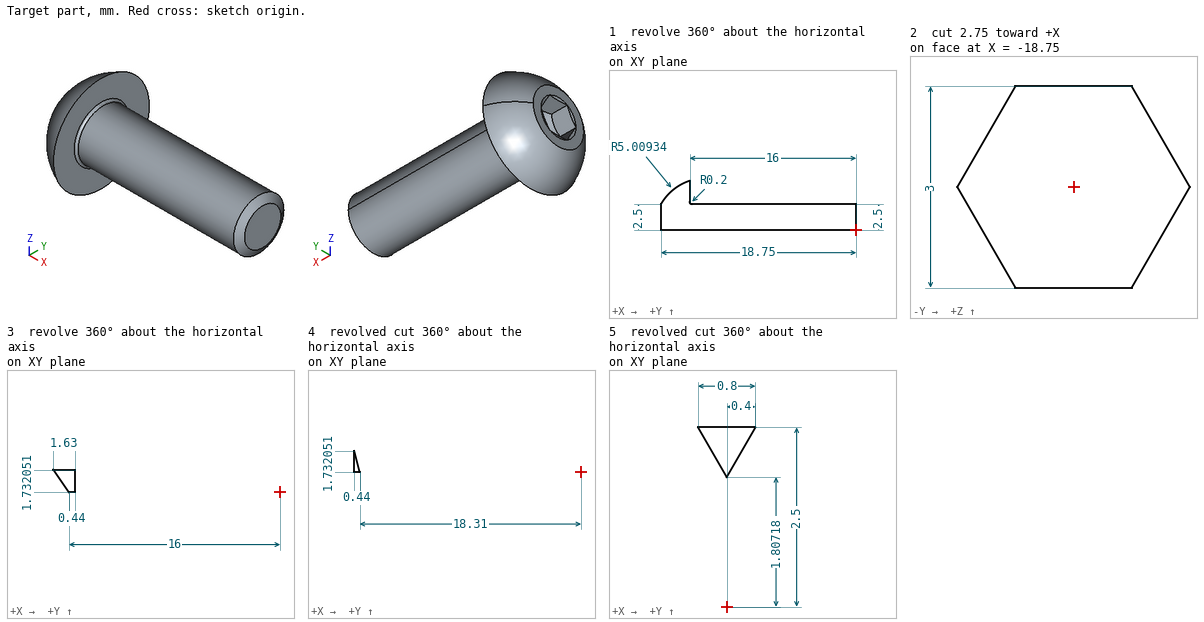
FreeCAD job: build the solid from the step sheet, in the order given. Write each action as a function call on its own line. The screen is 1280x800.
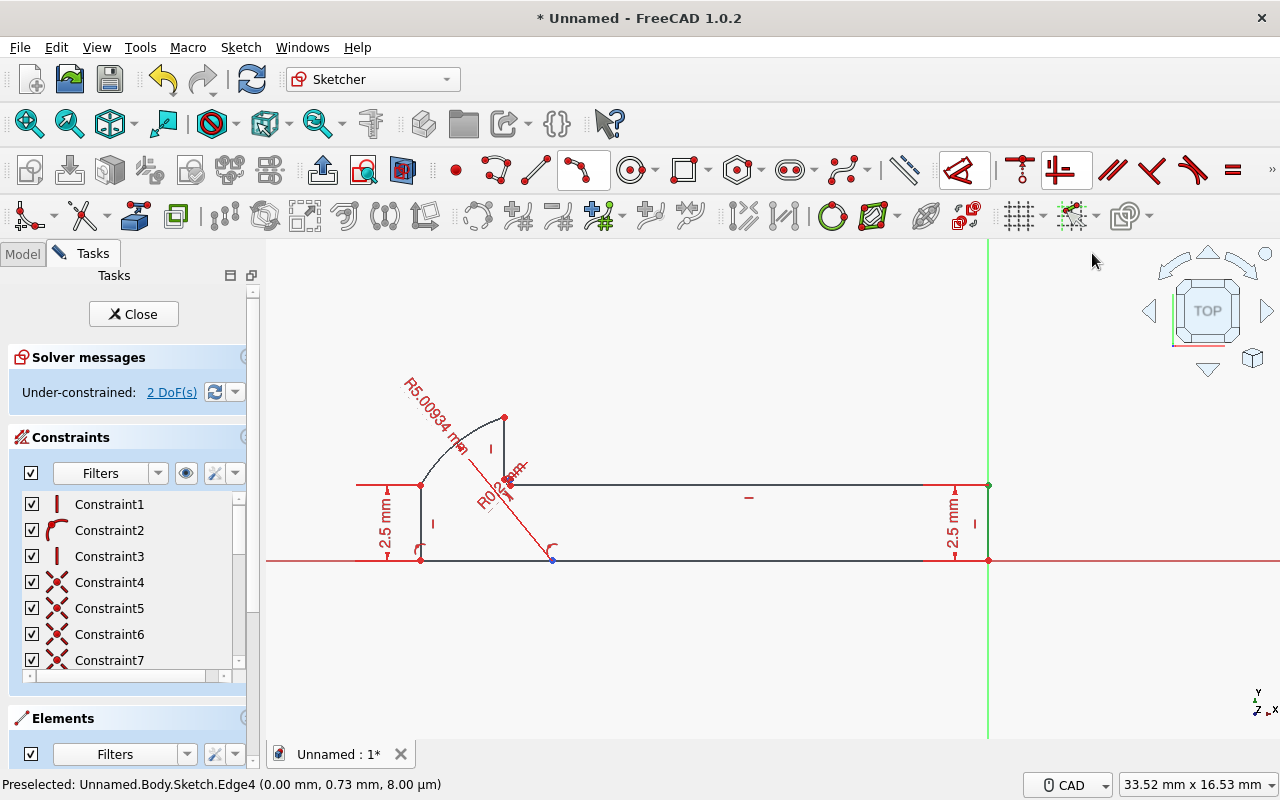
scroll(504, 479, up, 4)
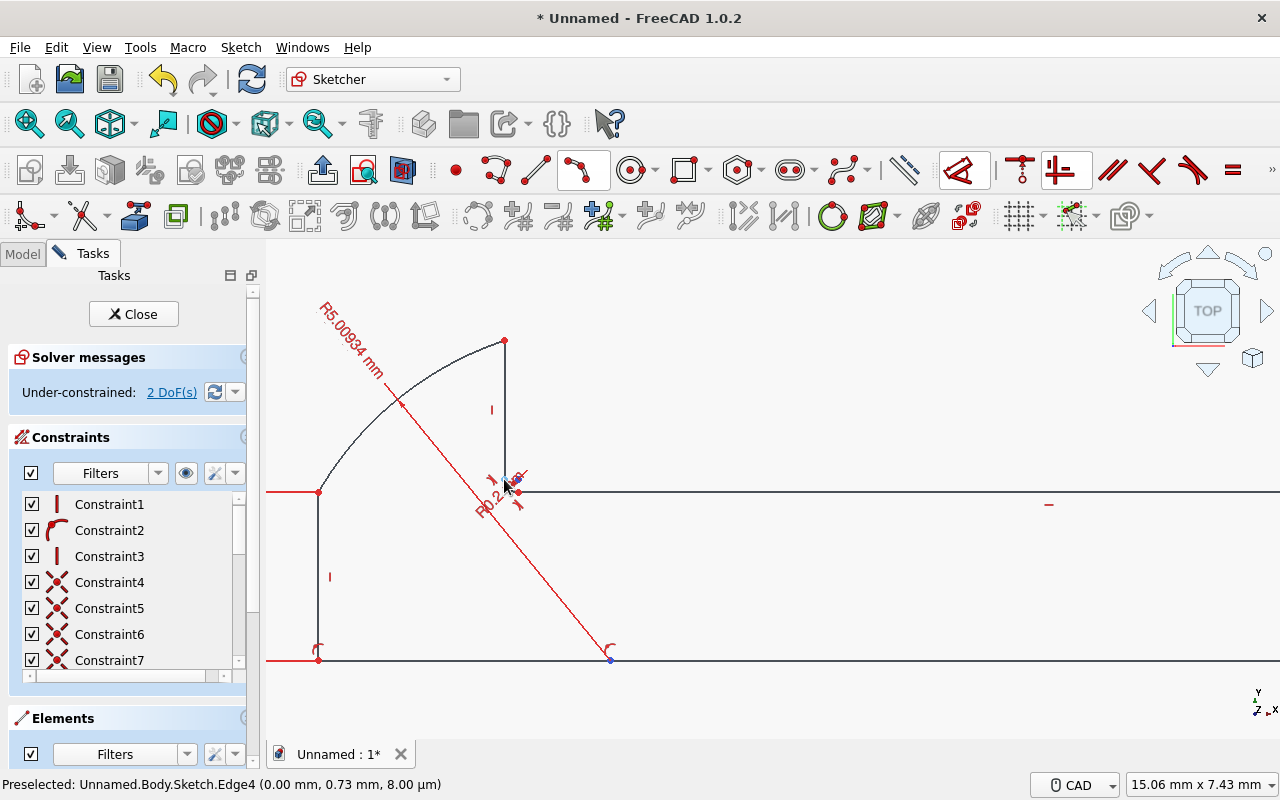
click(505, 479)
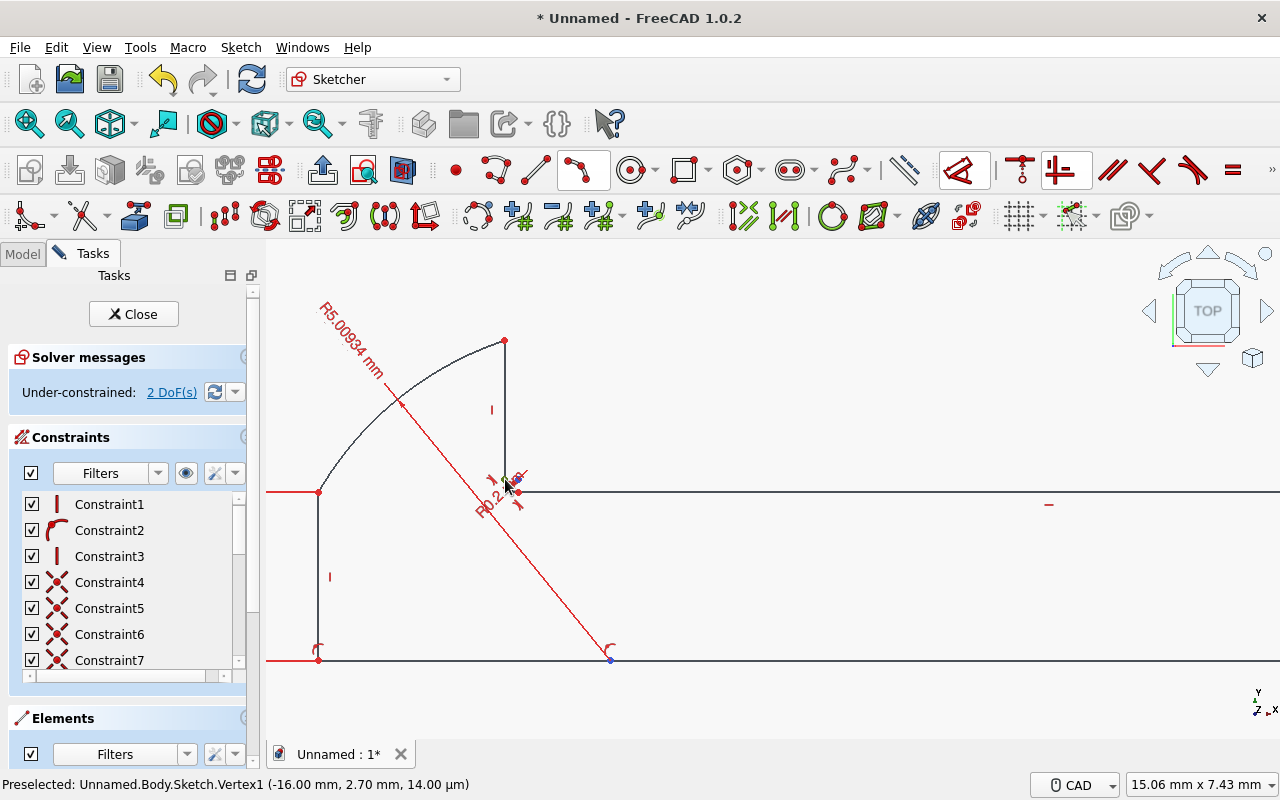
key(l)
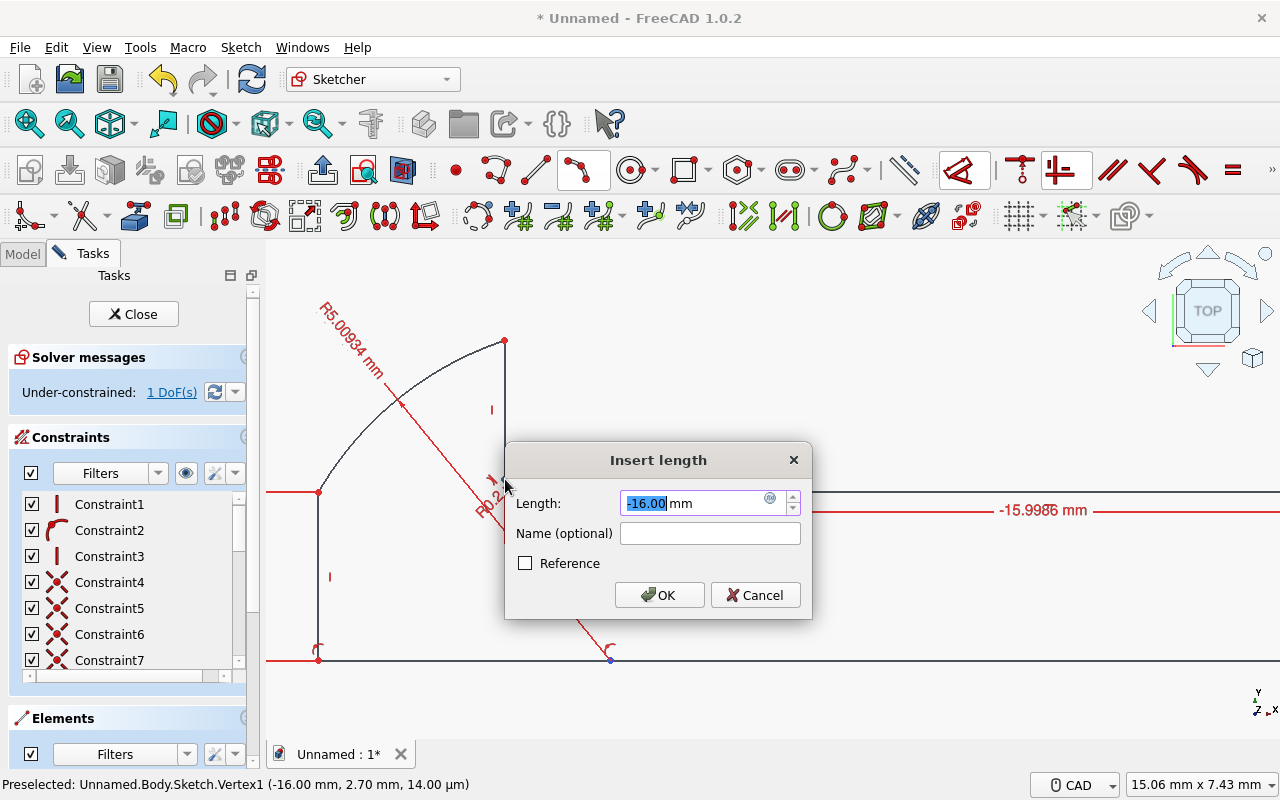
text(-16)
key(Return)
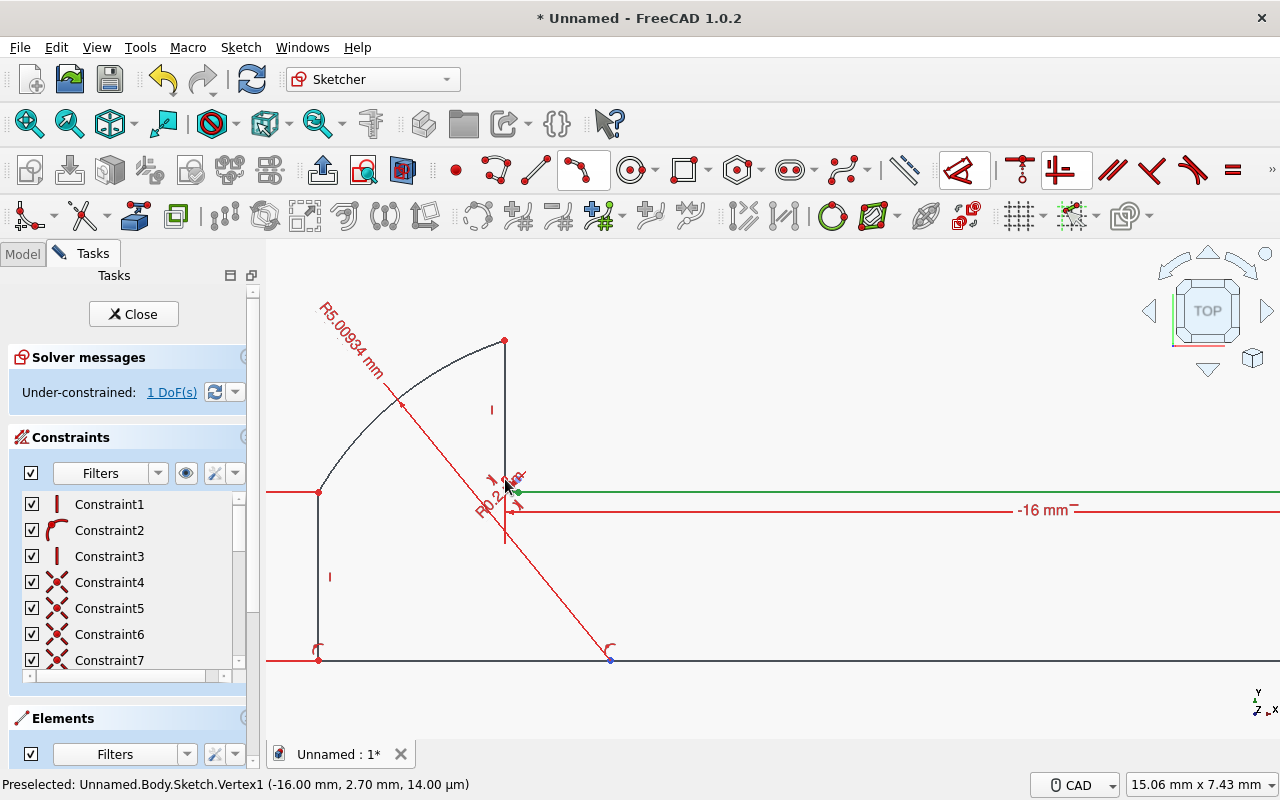
click(697, 661)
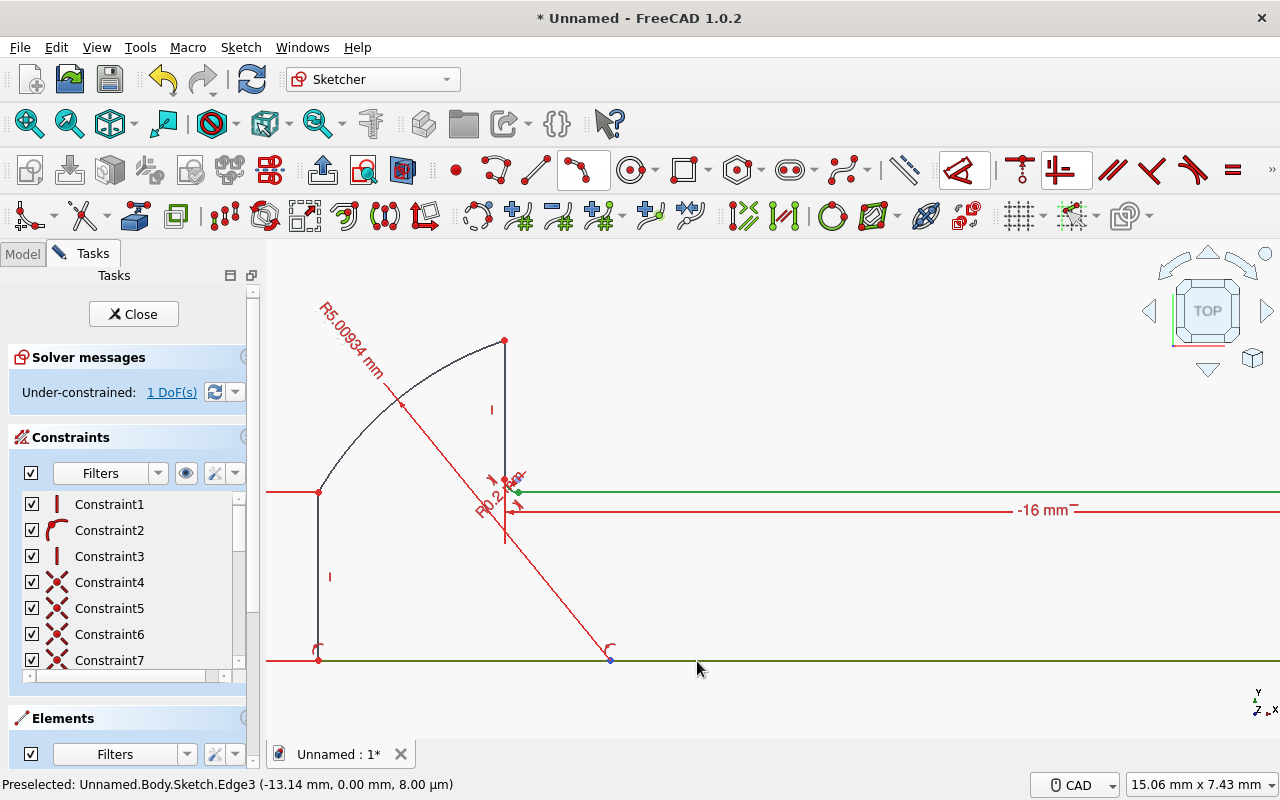
key(l)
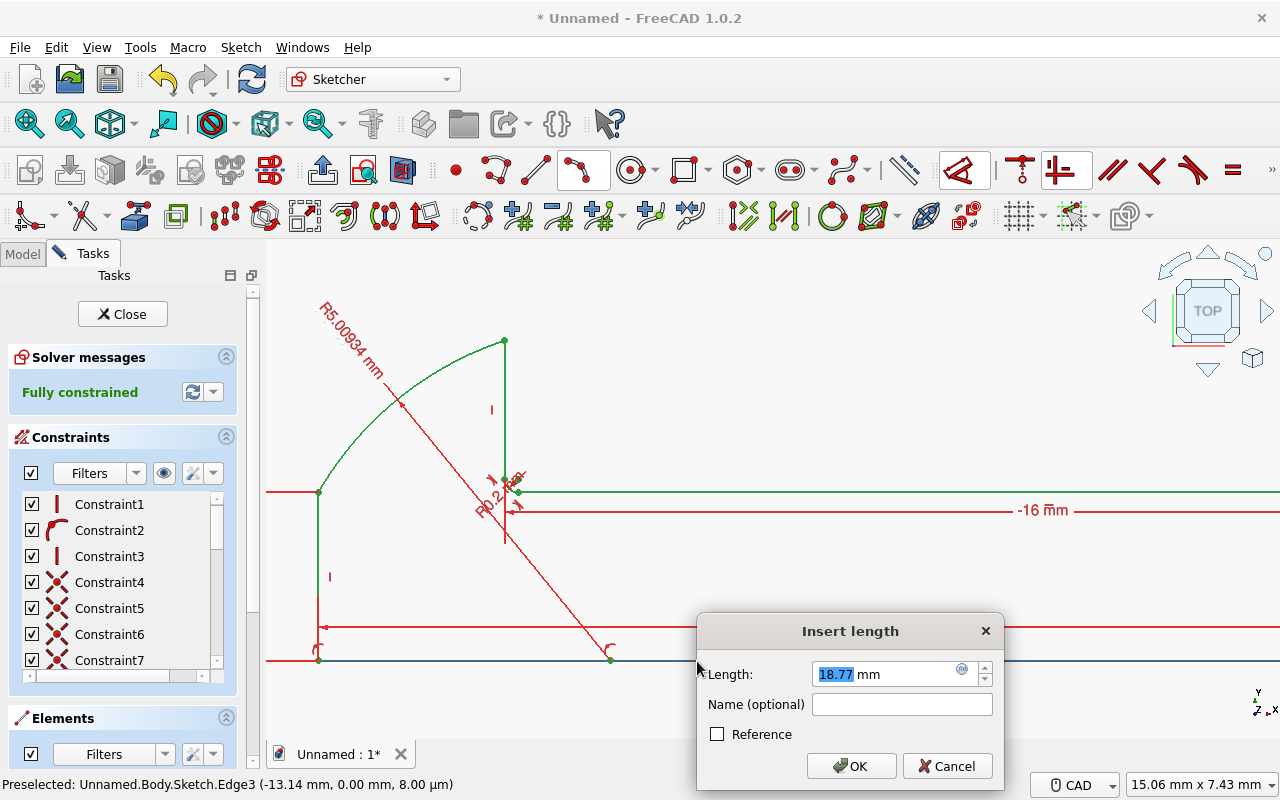
text(18.75)
key(Return)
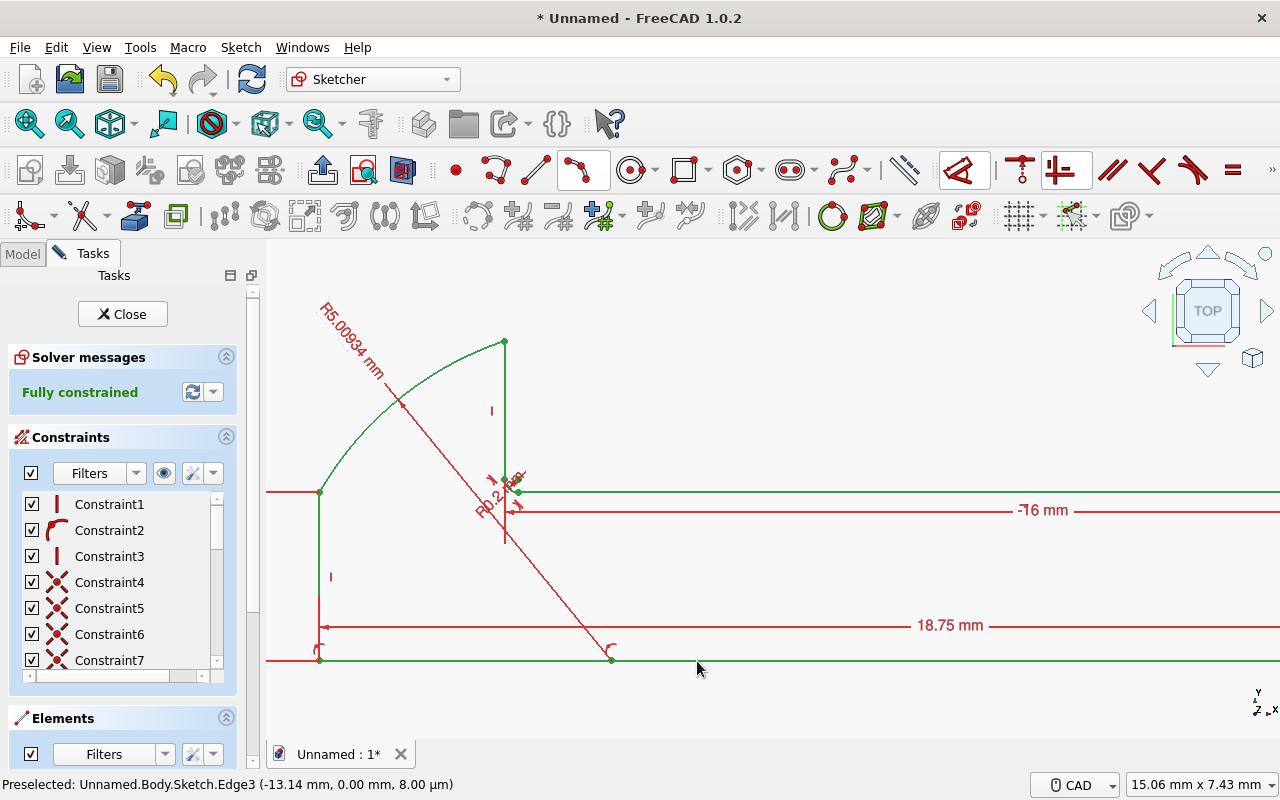
click(123, 314)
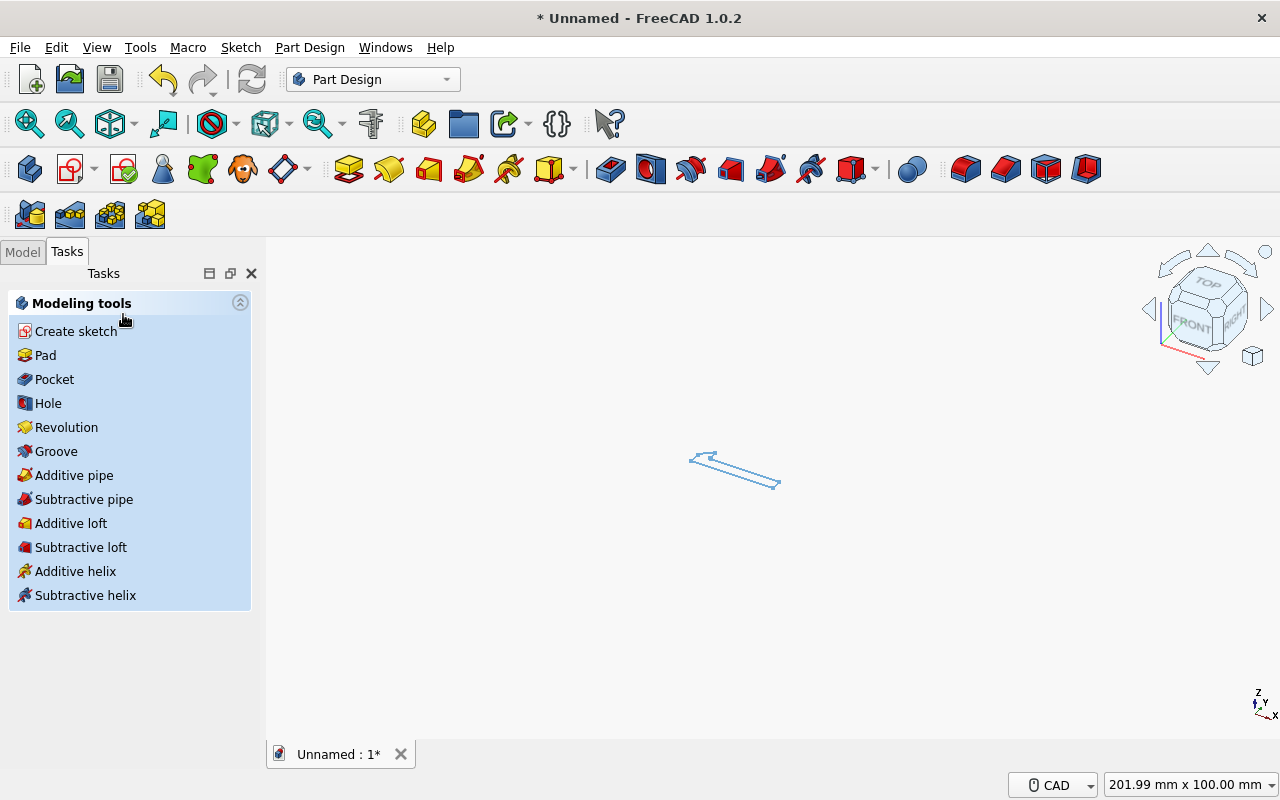
click(390, 170)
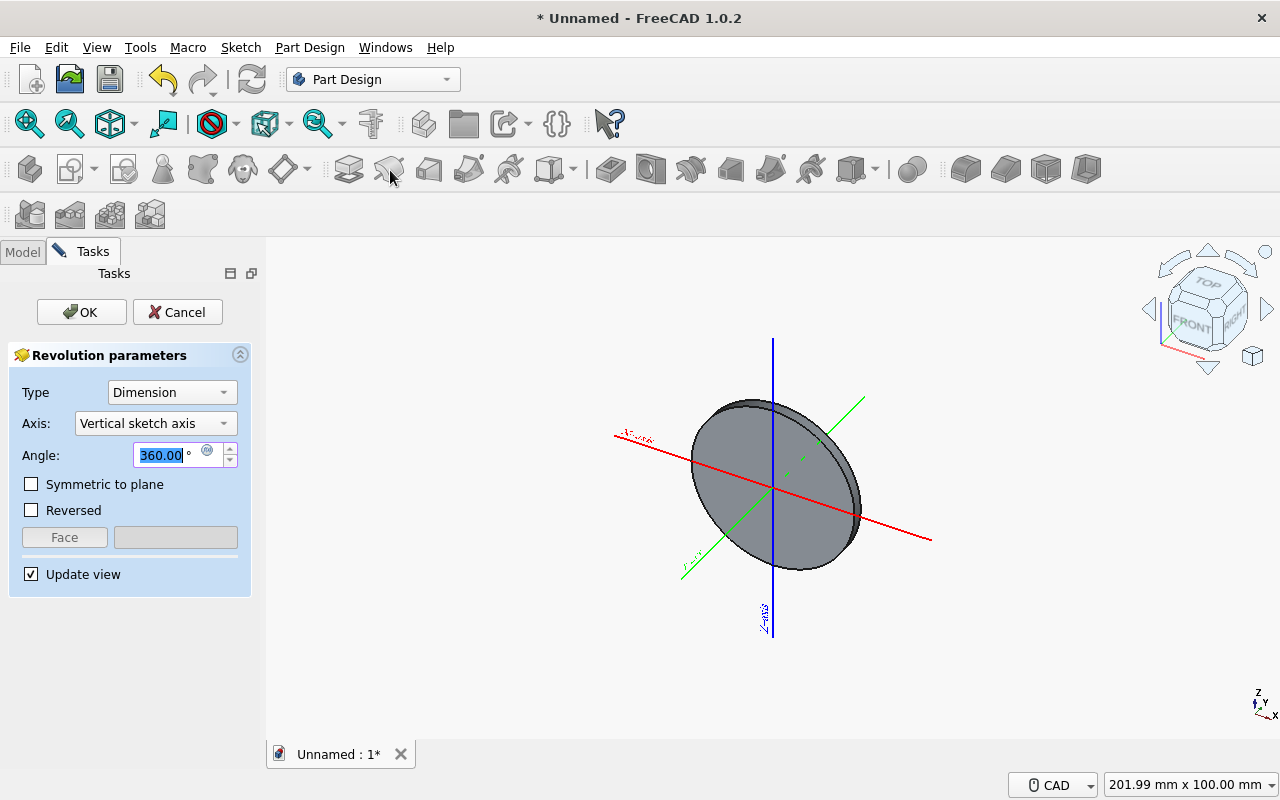
click(156, 424)